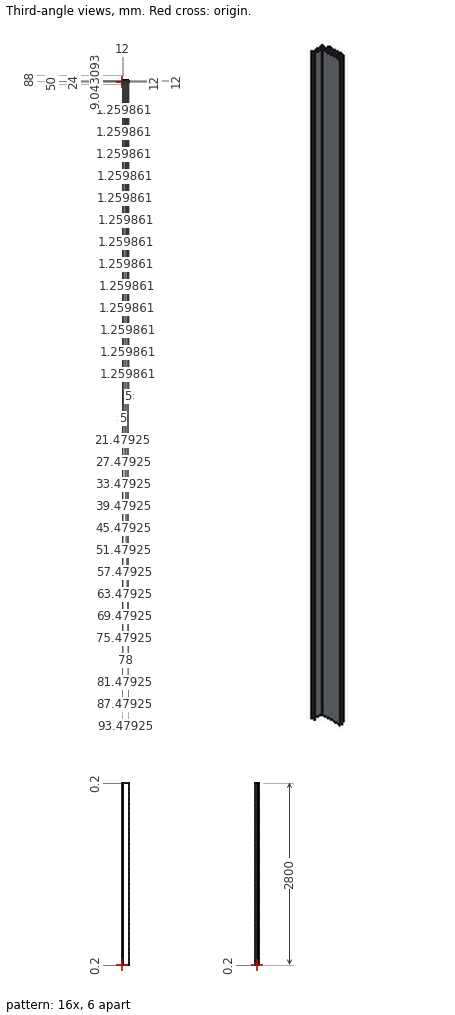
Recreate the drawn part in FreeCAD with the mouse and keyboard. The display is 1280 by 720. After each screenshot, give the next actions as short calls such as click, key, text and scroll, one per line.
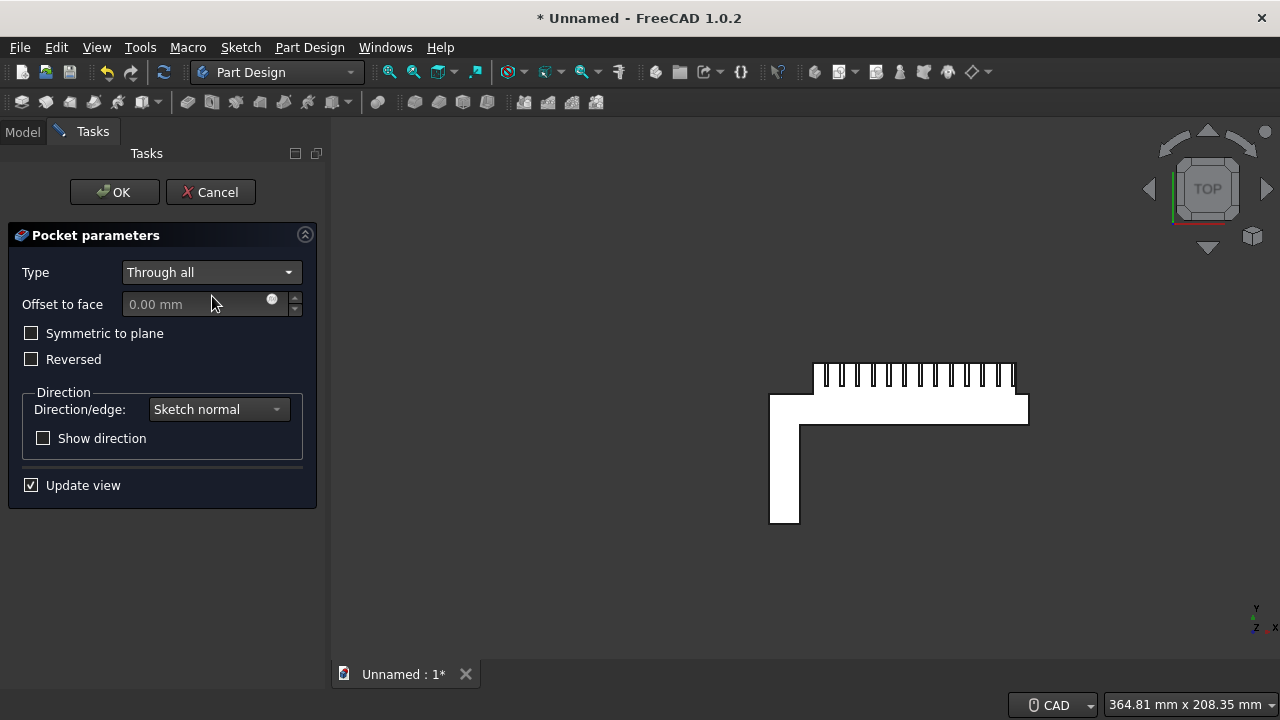
click(115, 192)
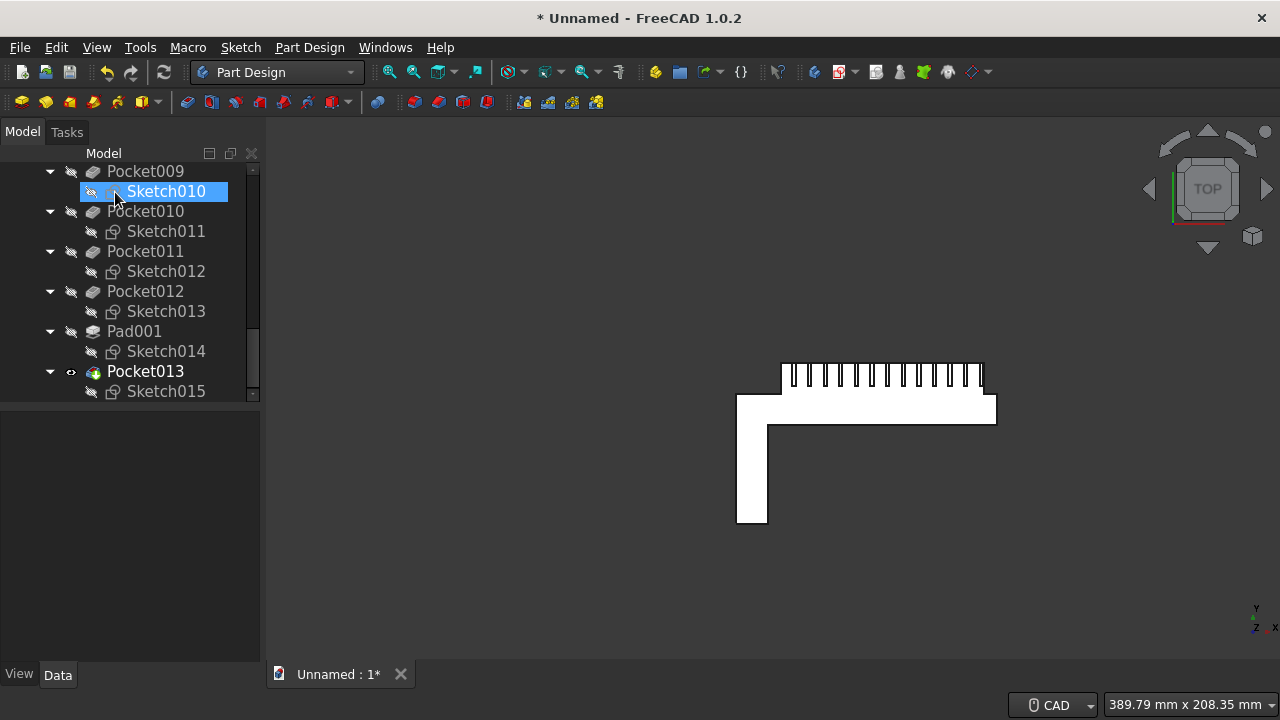
key(0)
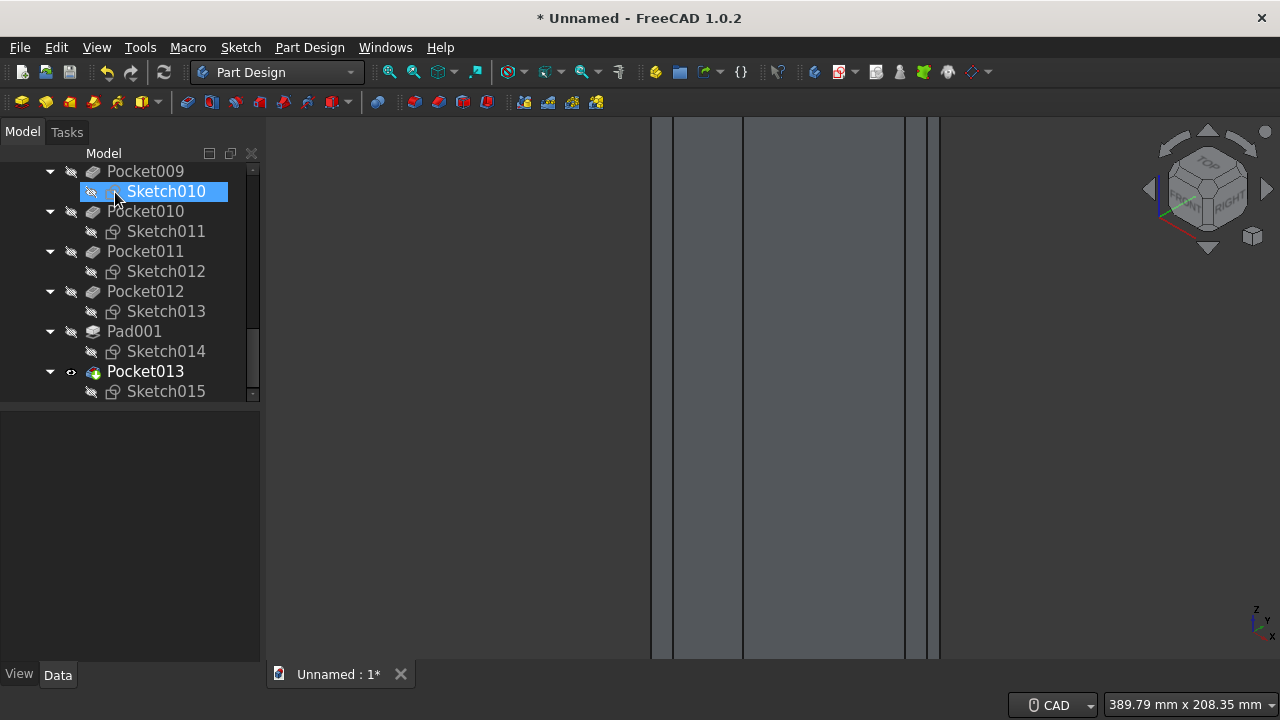
click(390, 72)